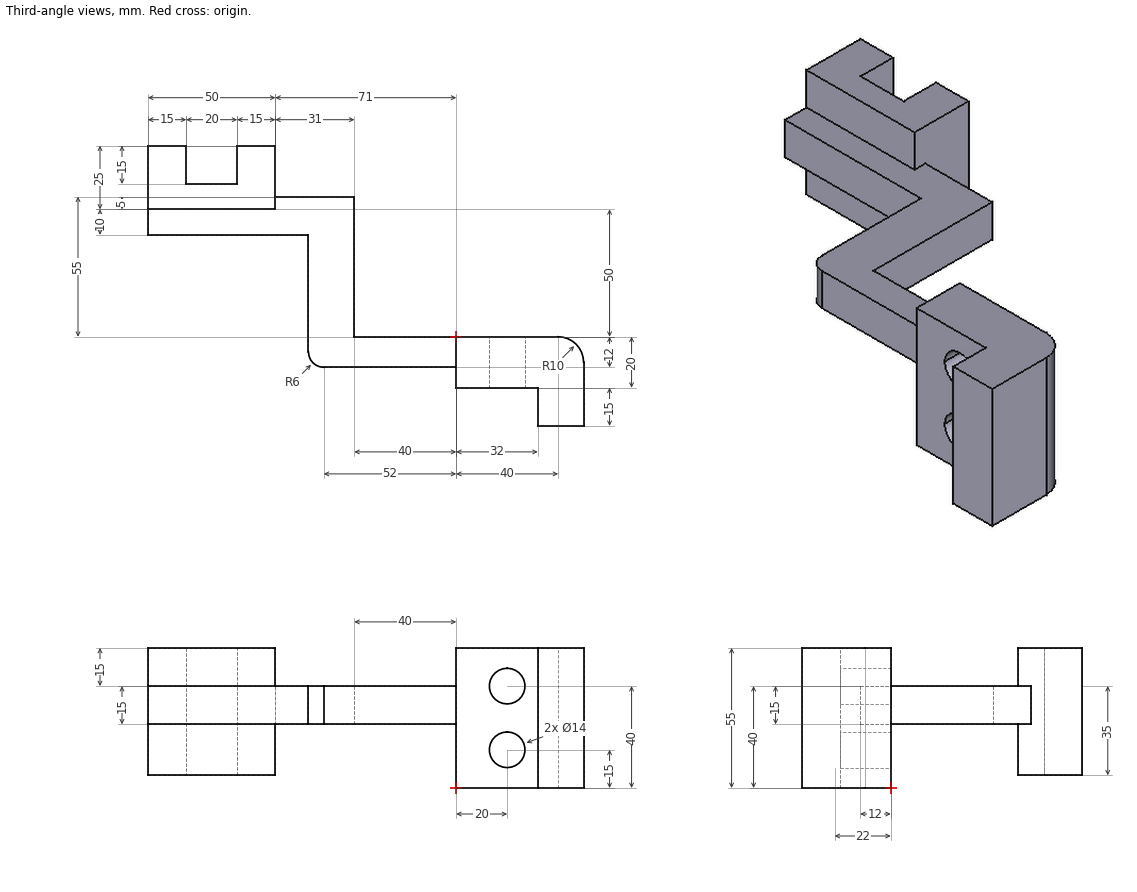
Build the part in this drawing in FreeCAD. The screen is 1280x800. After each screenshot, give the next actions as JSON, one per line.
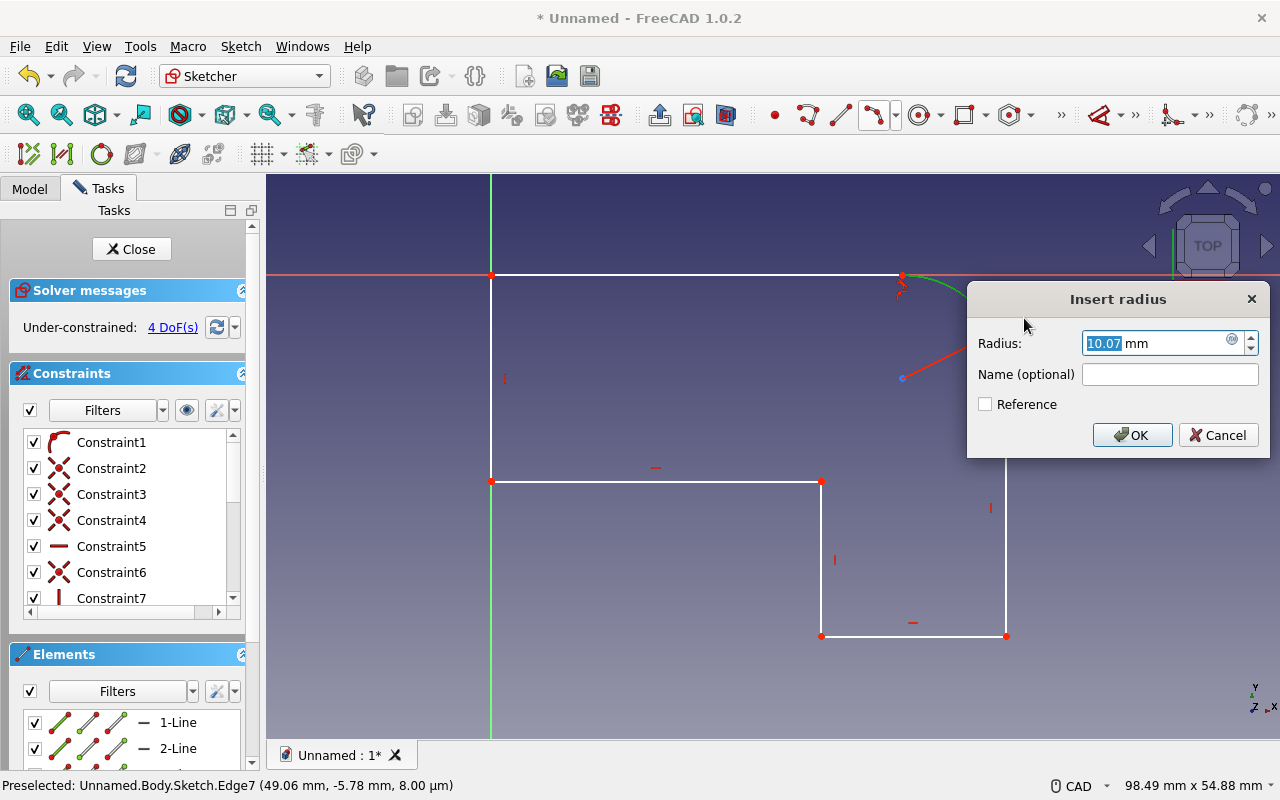
{"action": "type", "text": "10"}
{"action": "key", "text": "Return"}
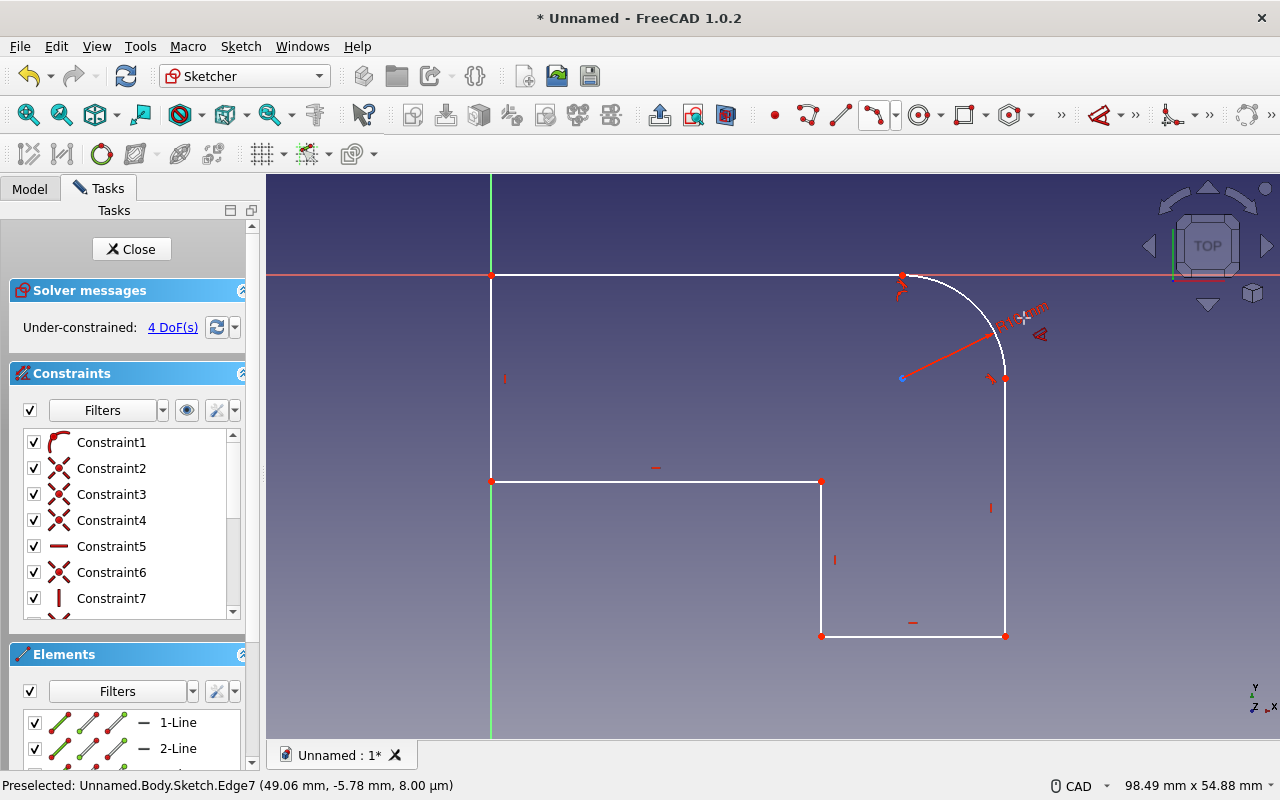
{"action": "left_click", "coordinate": [779, 275]}
{"action": "left_click", "coordinate": [697, 241]}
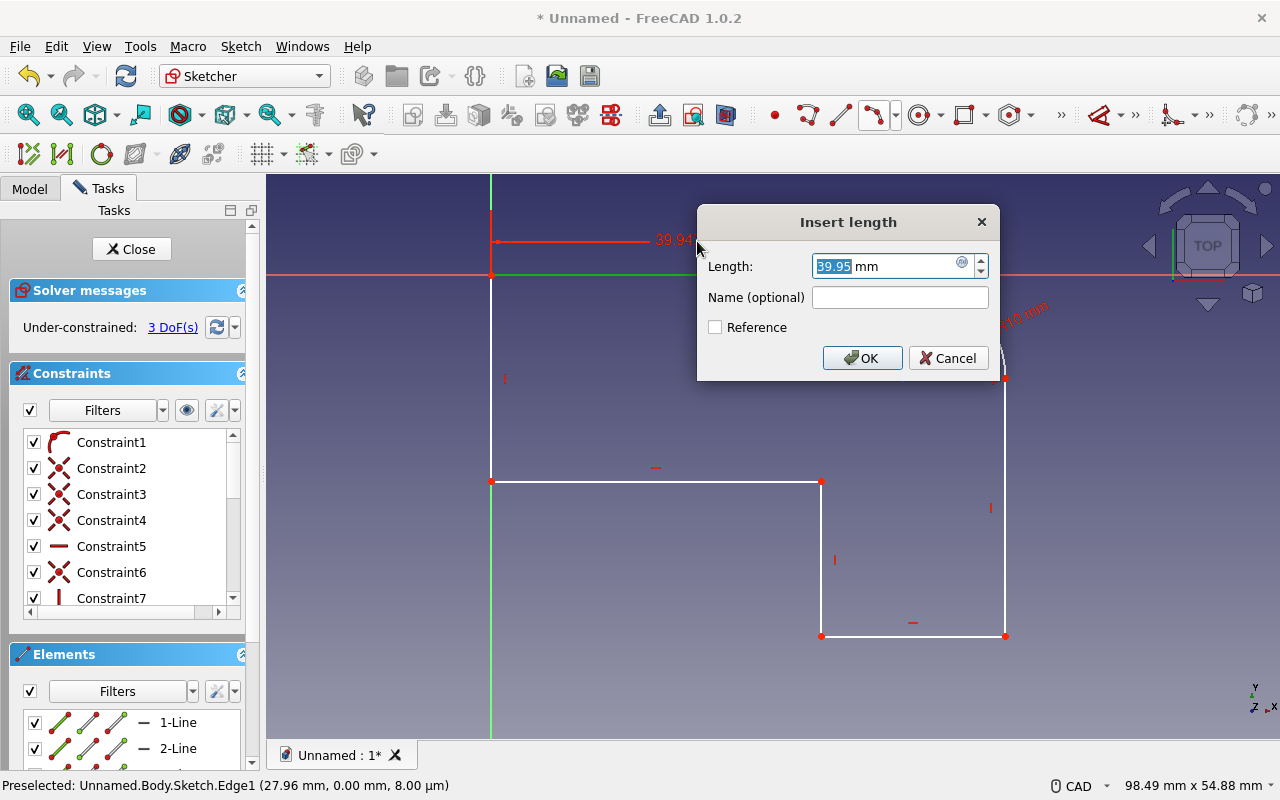
{"action": "type", "text": "40"}
{"action": "key", "text": "Return"}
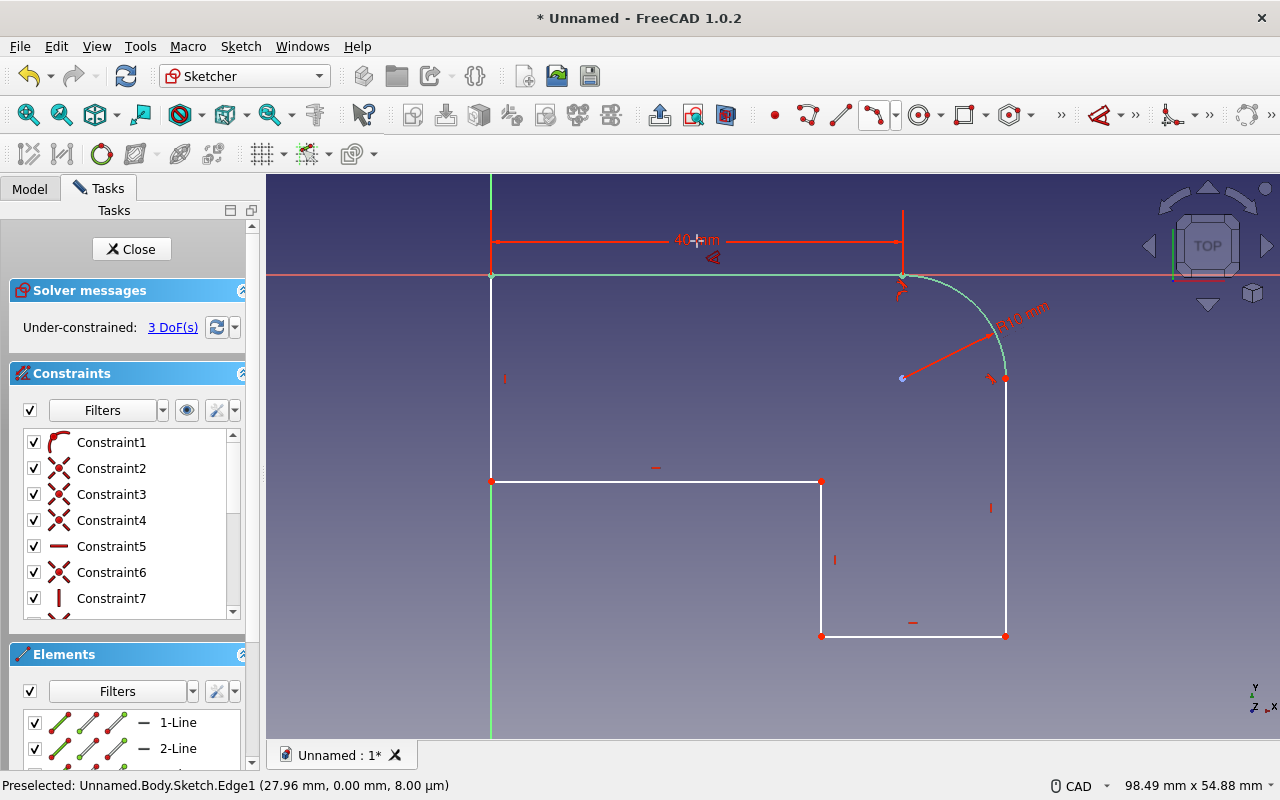
{"action": "left_click", "coordinate": [491, 337]}
{"action": "left_click", "coordinate": [457, 379]}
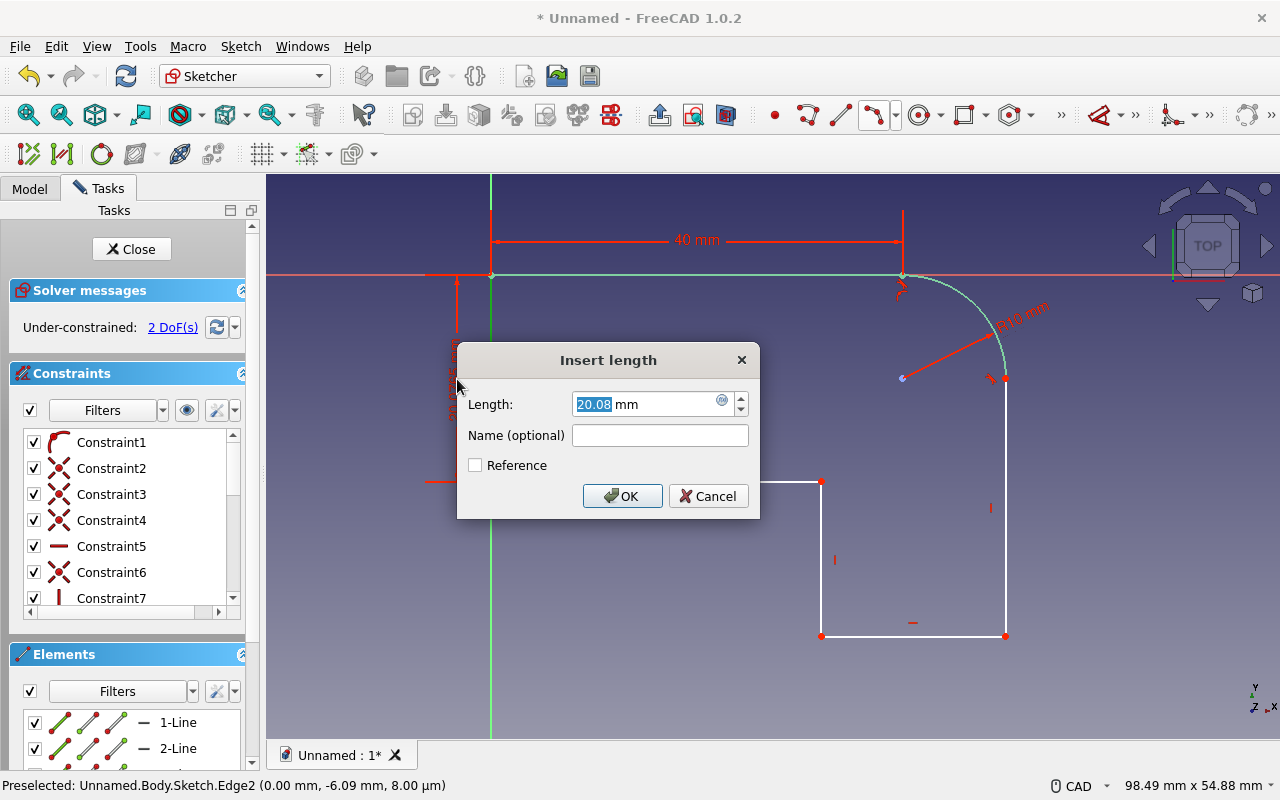
{"action": "type", "text": "20"}
{"action": "key", "text": "Return"}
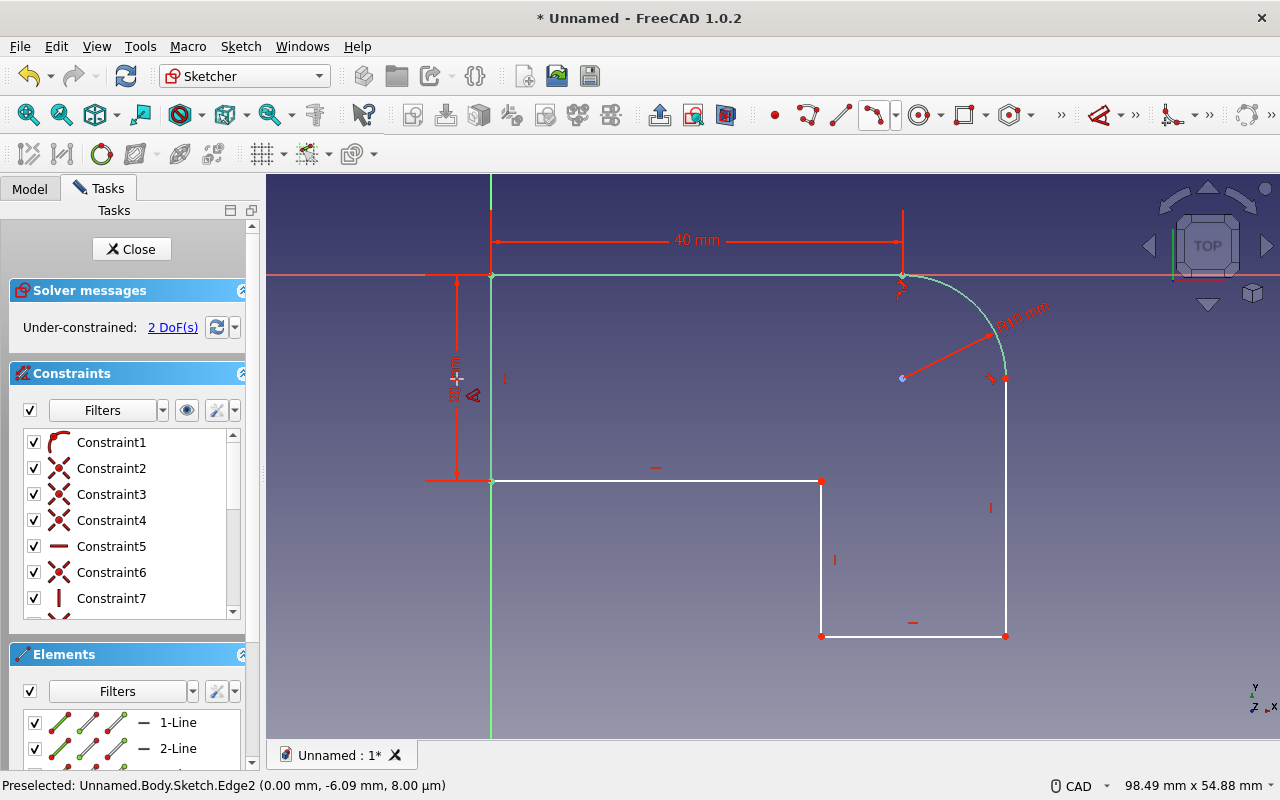
{"action": "left_click", "coordinate": [590, 481]}
{"action": "left_click", "coordinate": [656, 515]}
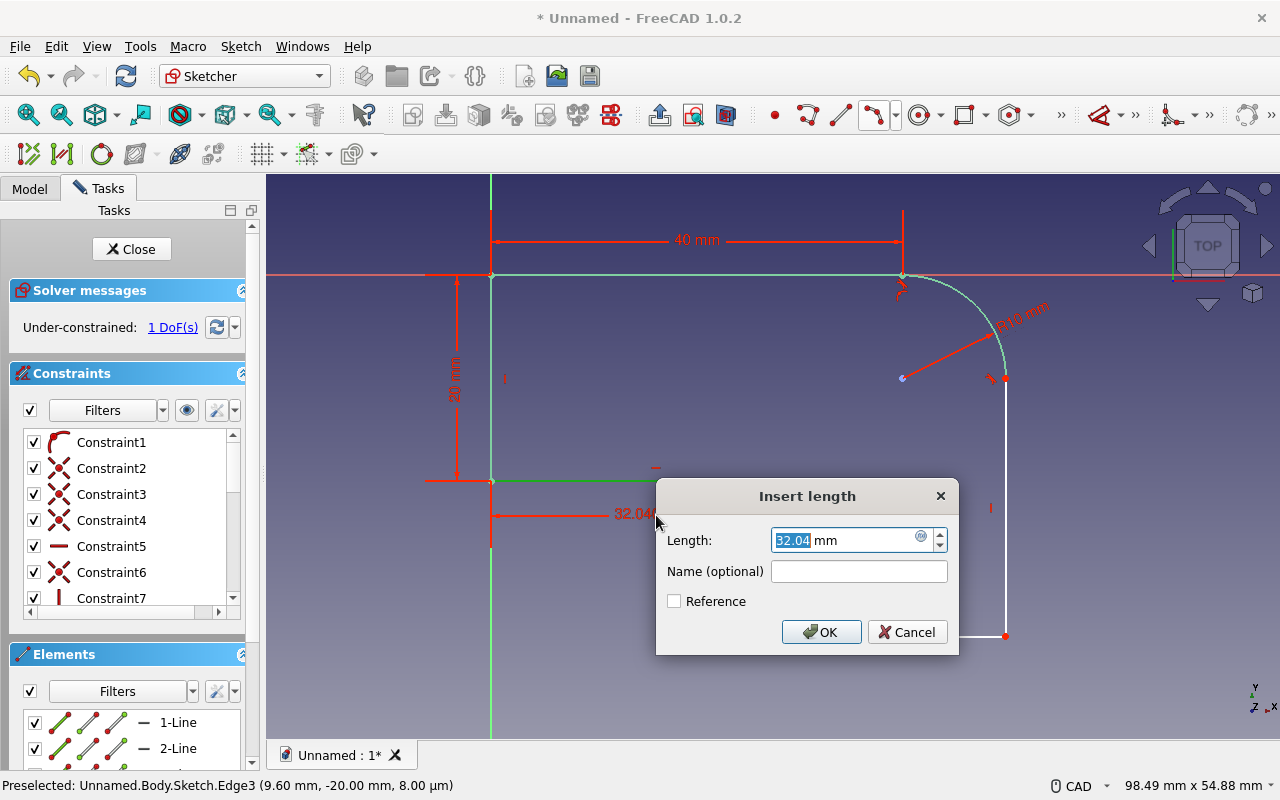
{"action": "type", "text": "32"}
{"action": "key", "text": "Return"}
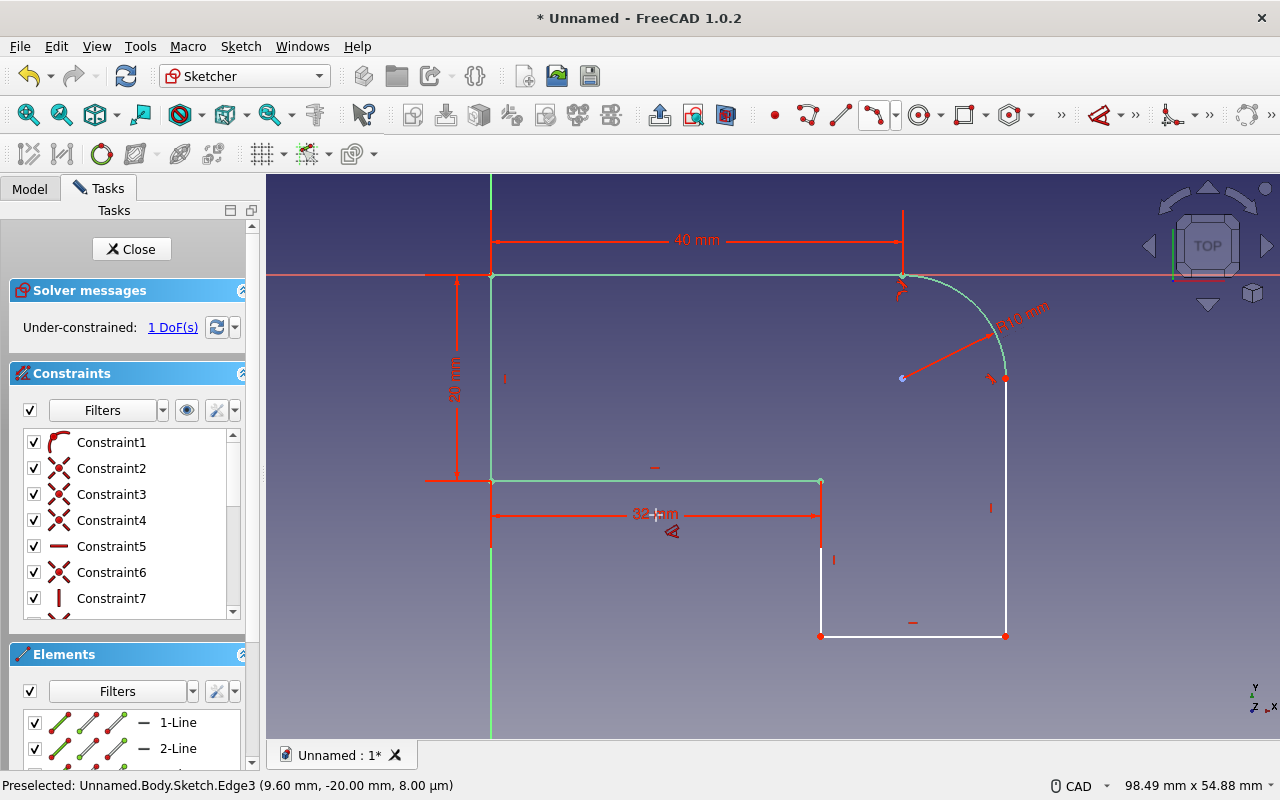
{"action": "left_click", "coordinate": [821, 528]}
{"action": "left_click", "coordinate": [855, 559]}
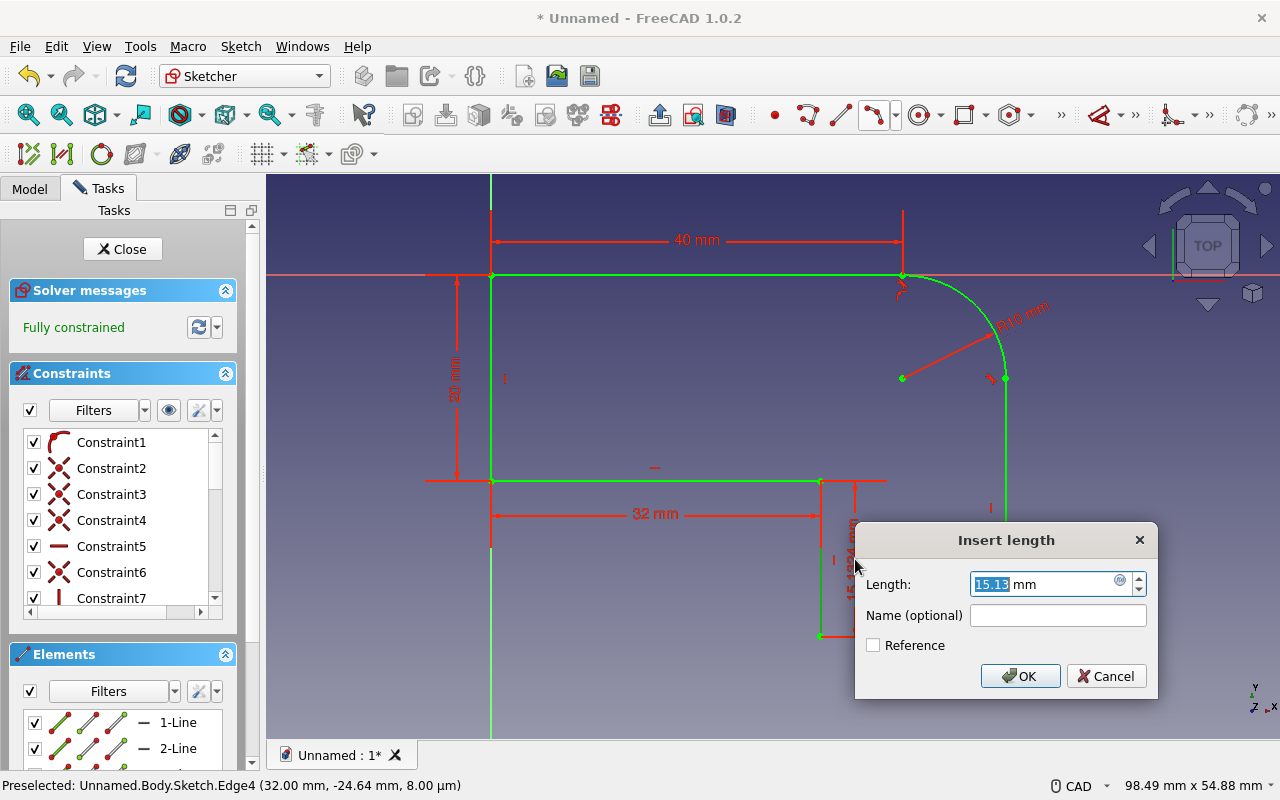
{"action": "type", "text": "15"}
{"action": "key", "text": "Return"}
{"action": "key", "text": "Escape"}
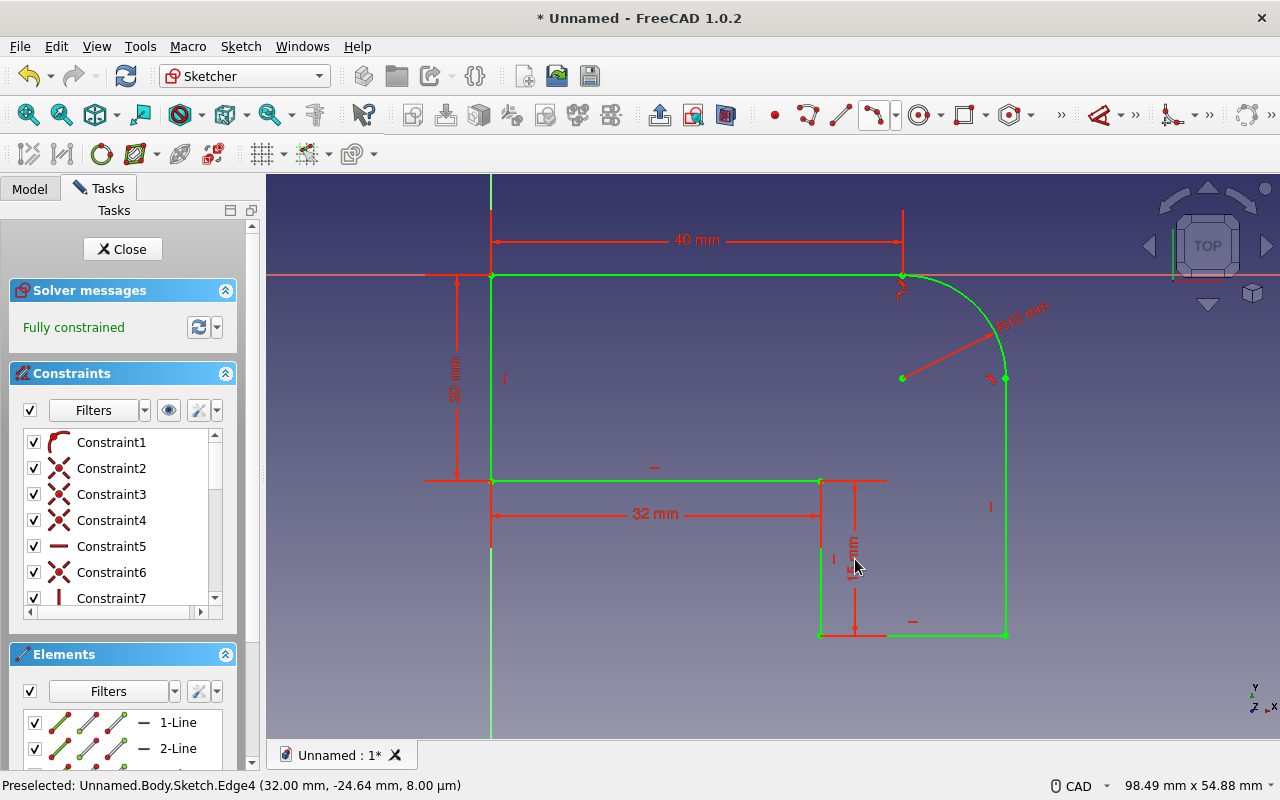
{"action": "left_click", "coordinate": [123, 249]}